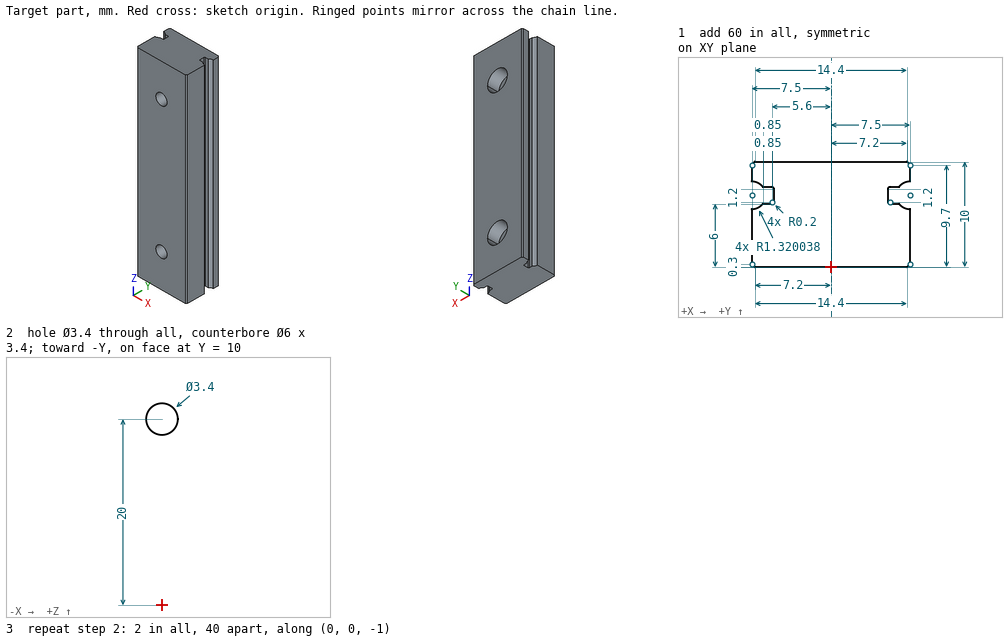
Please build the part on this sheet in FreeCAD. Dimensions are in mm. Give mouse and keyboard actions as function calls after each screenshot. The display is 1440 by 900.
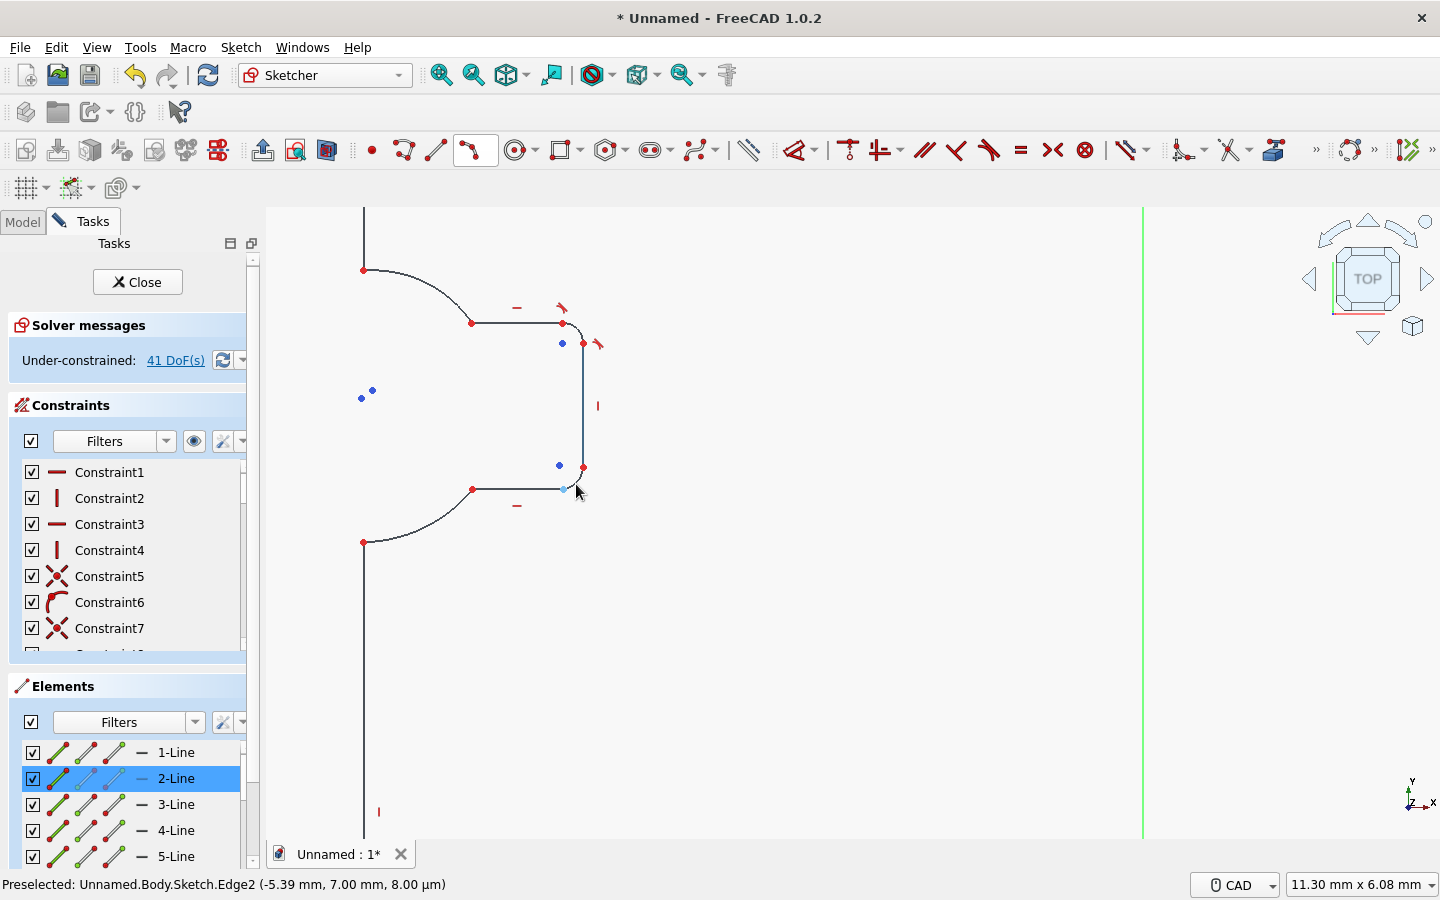
click(577, 482)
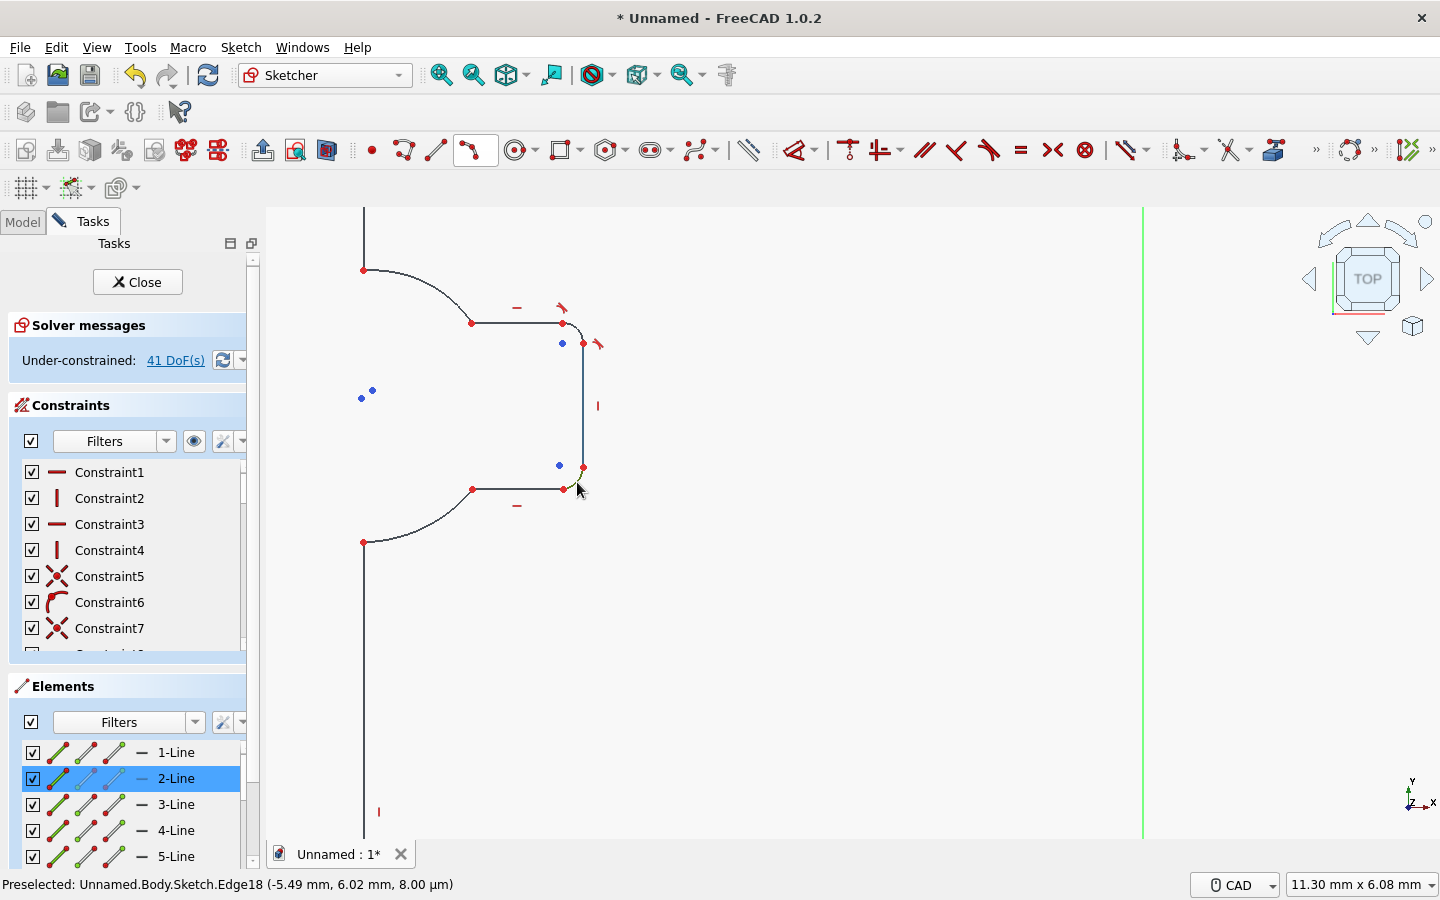
click(990, 150)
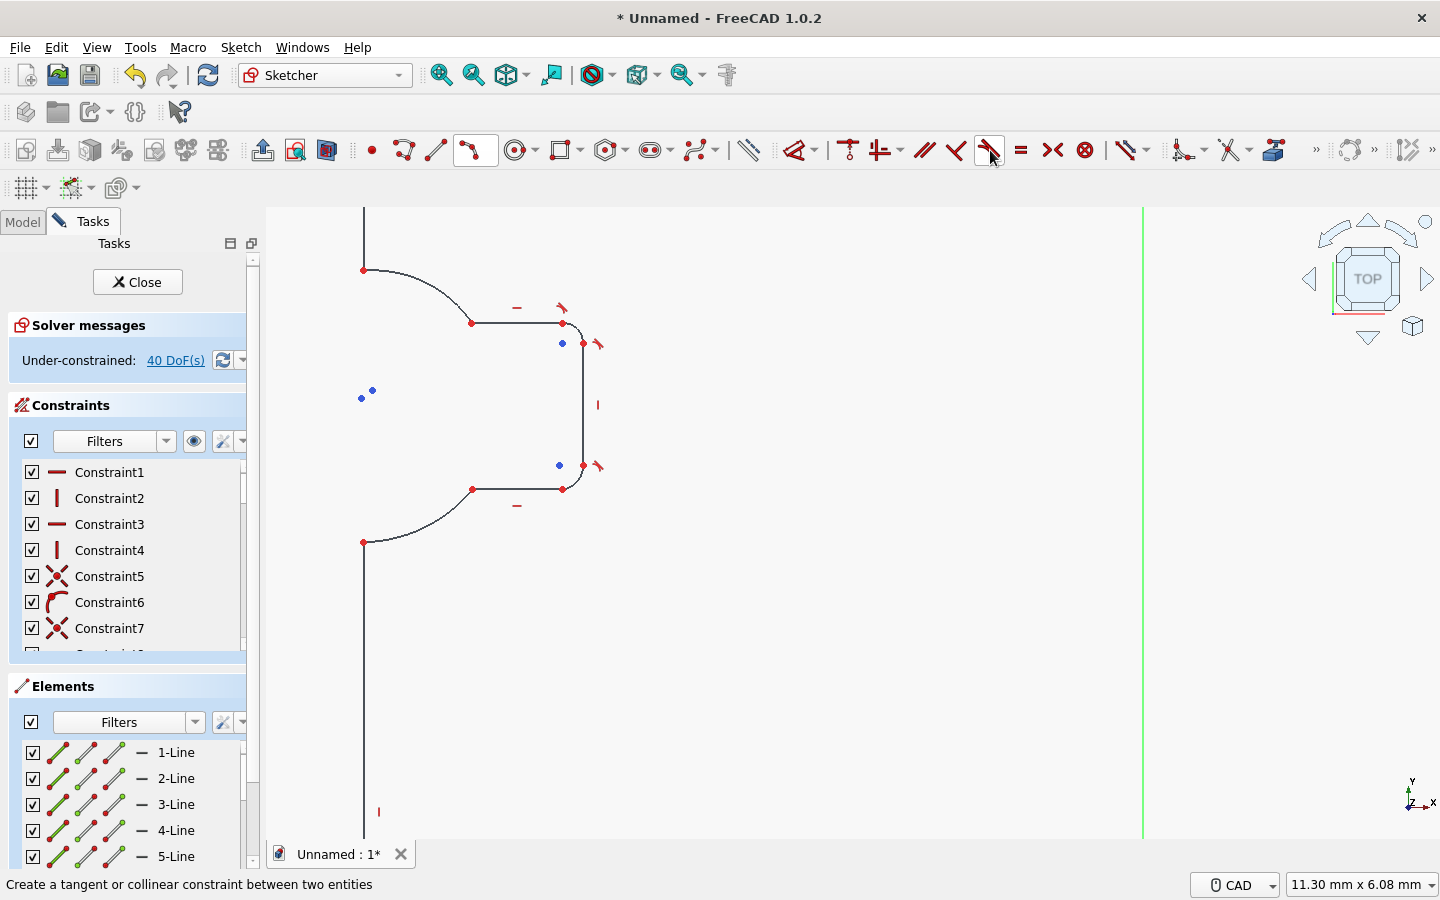
click(536, 489)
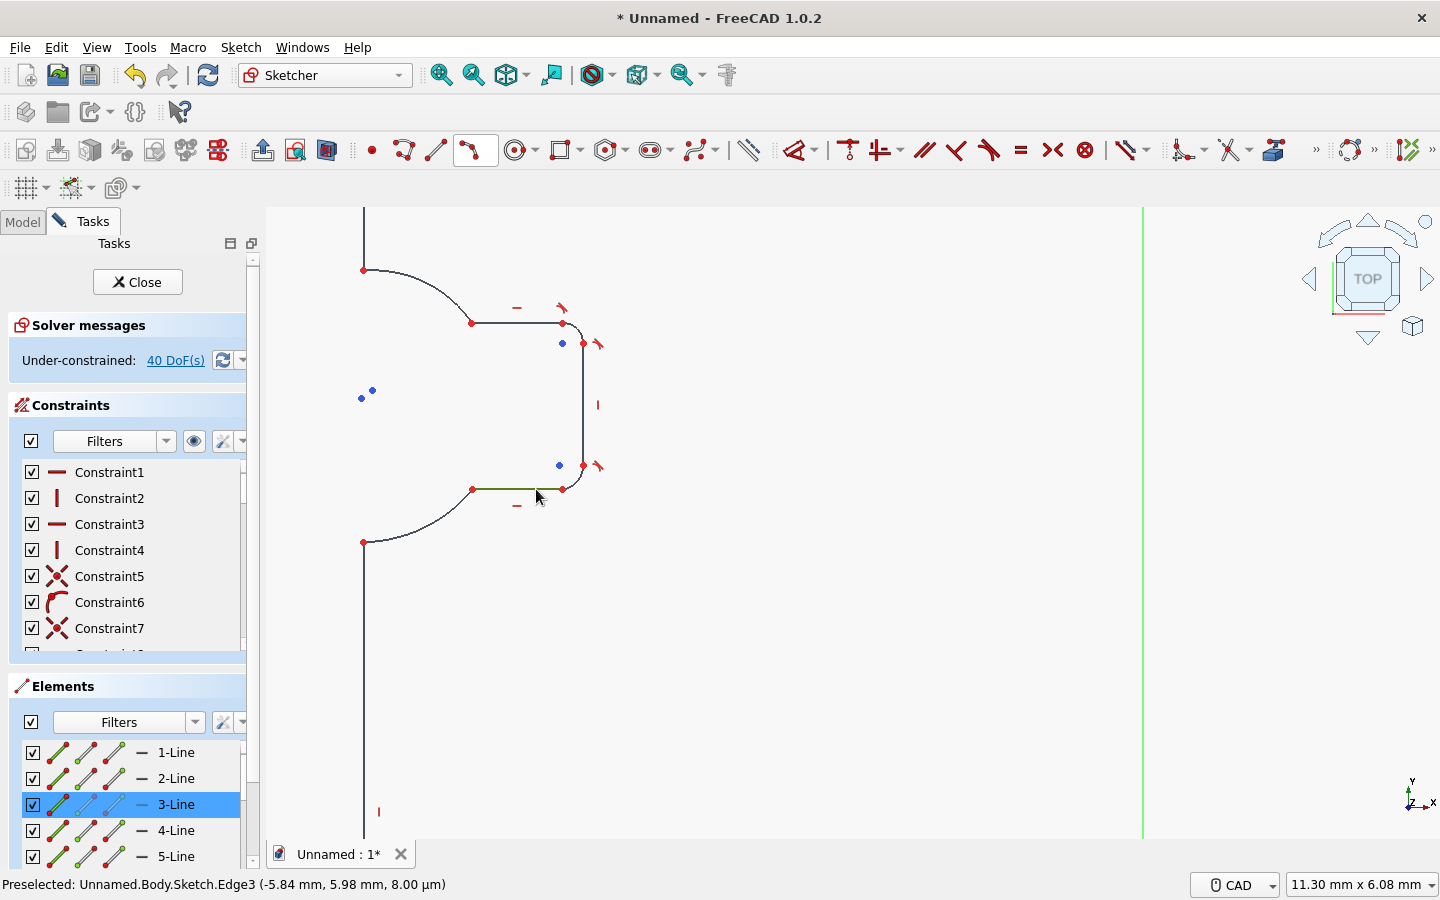
scroll(572, 486, up, 2)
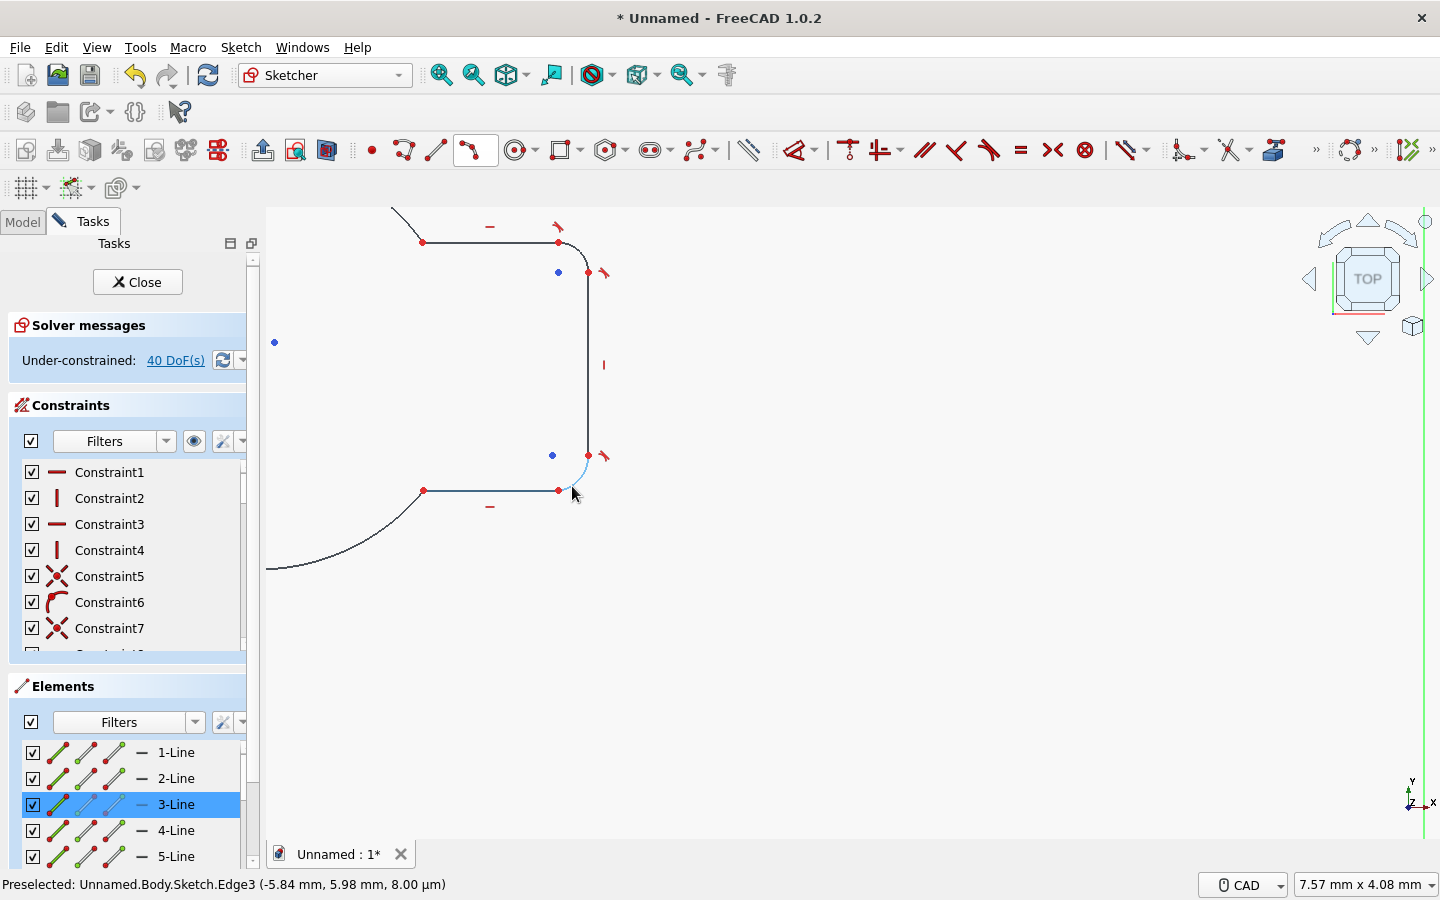
click(572, 486)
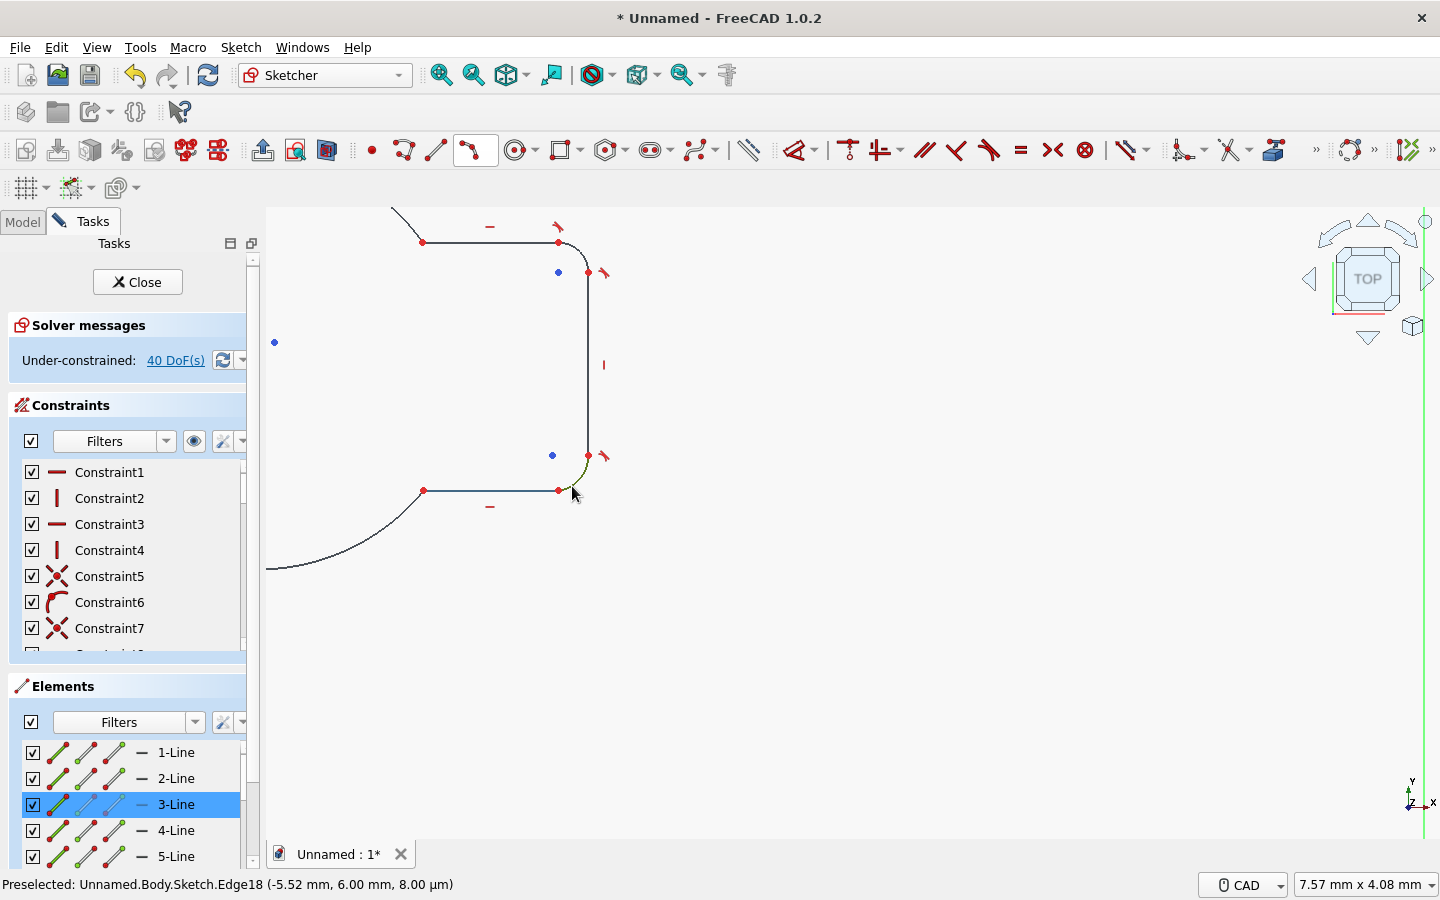
click(990, 150)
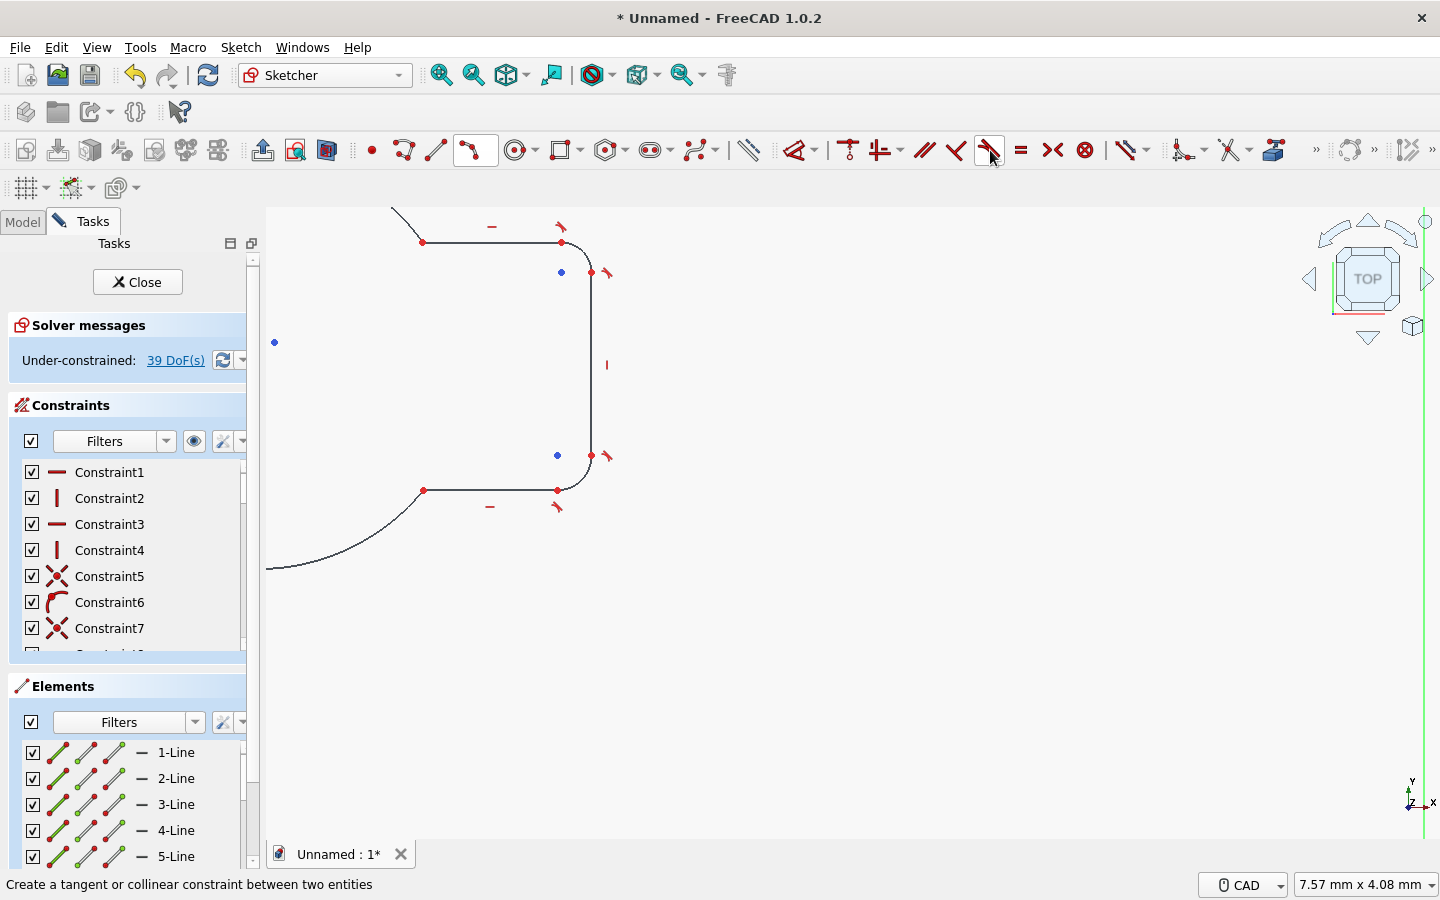
scroll(575, 484, down, 7)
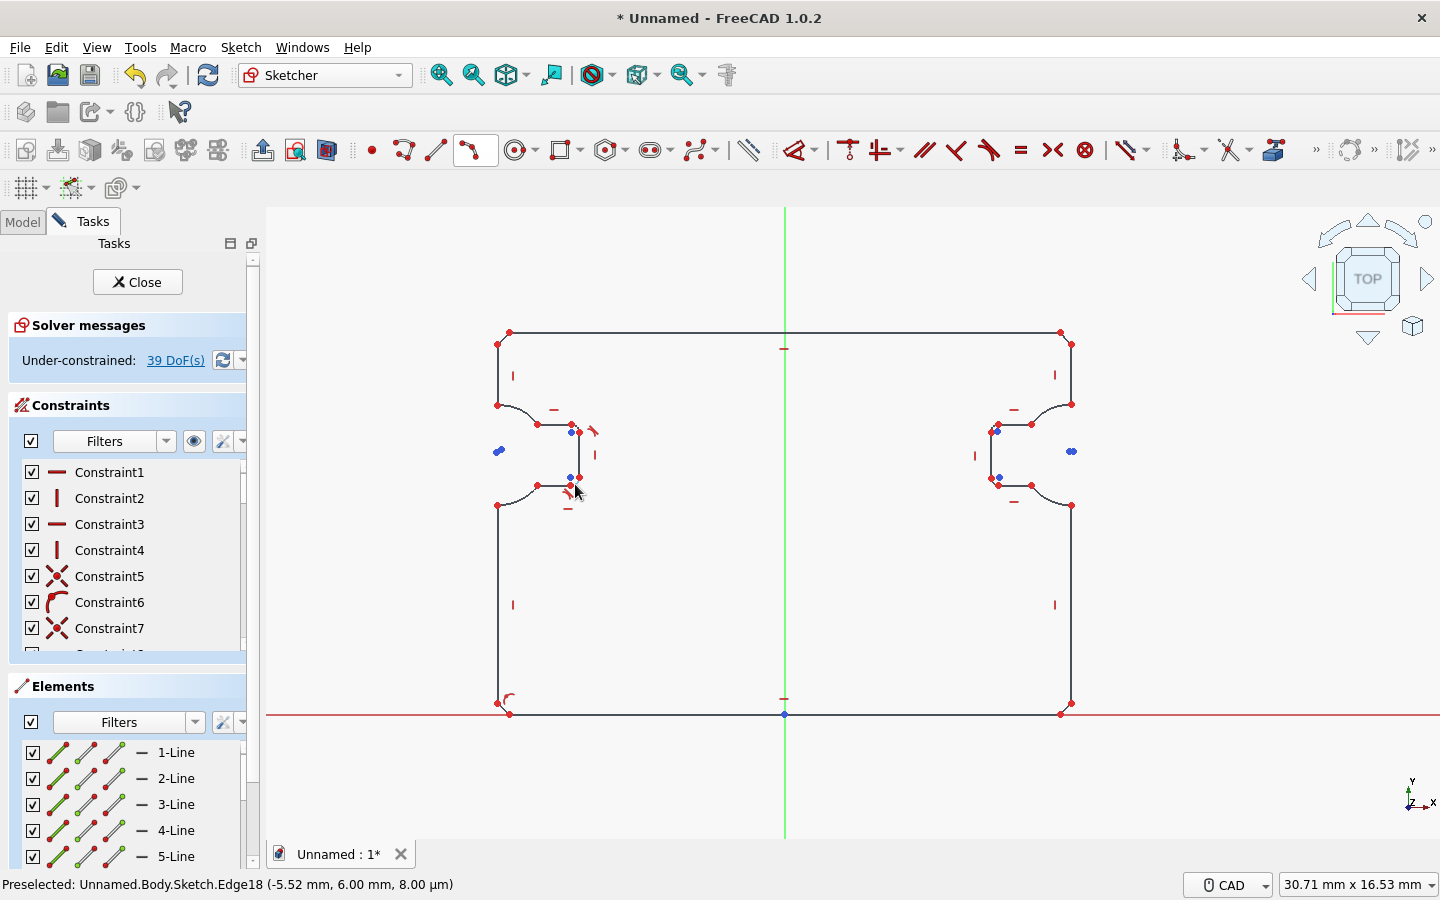
scroll(1021, 486, up, 2)